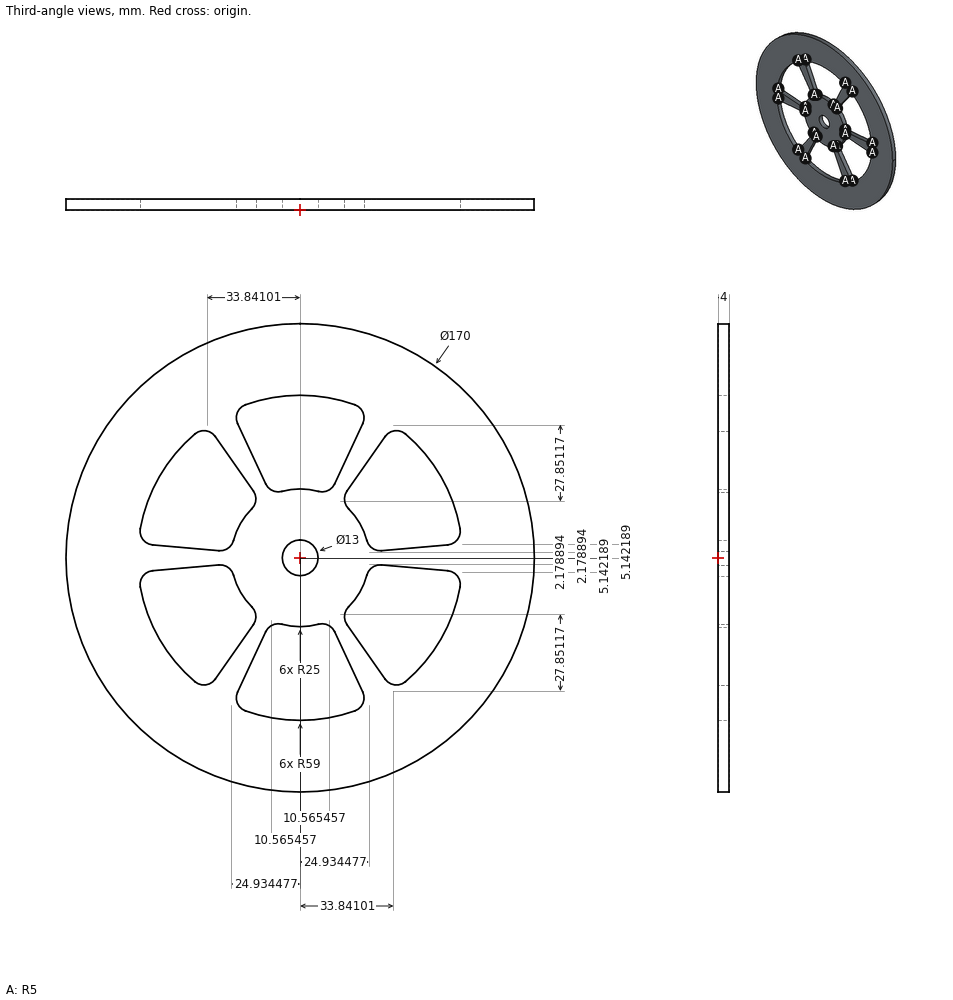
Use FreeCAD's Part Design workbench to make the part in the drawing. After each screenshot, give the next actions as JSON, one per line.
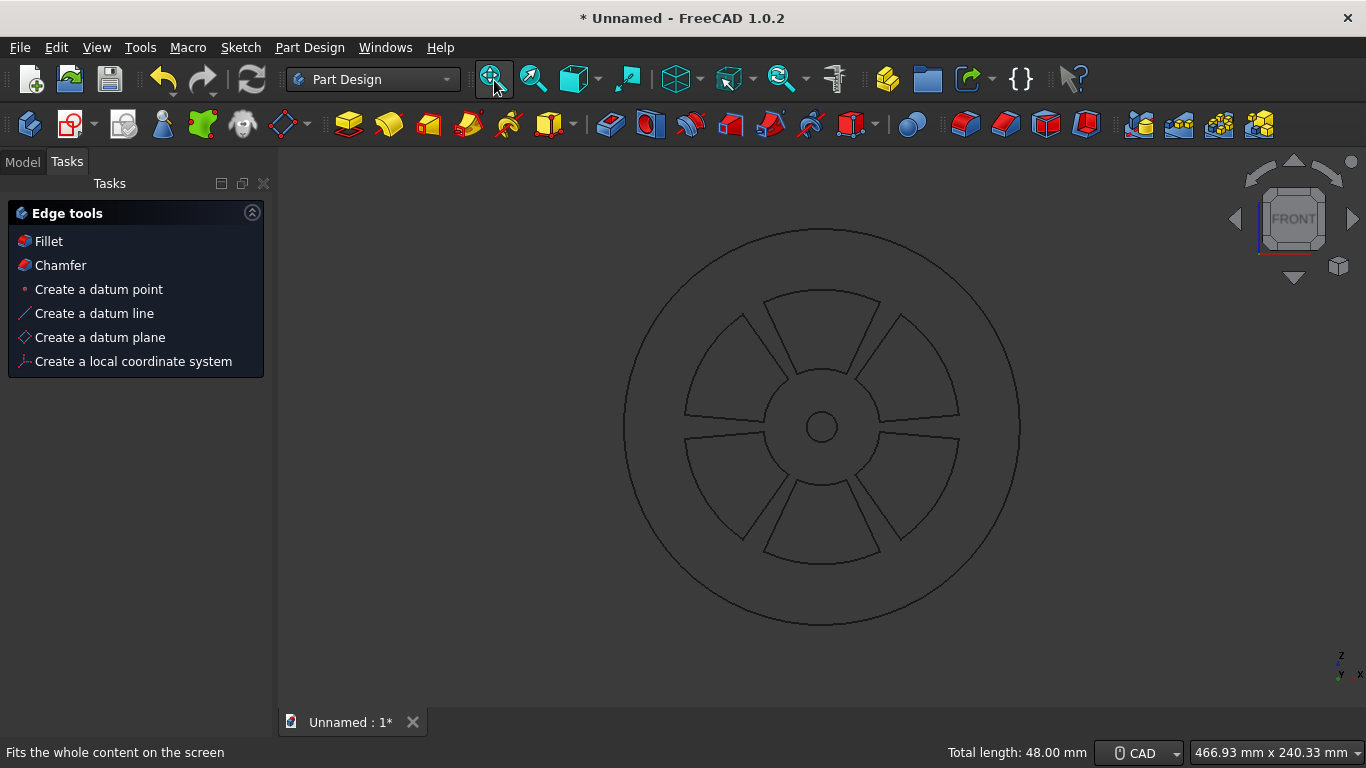
{"action": "scroll", "coordinate": [880, 421], "scroll_direction": "up", "scroll_amount": 8}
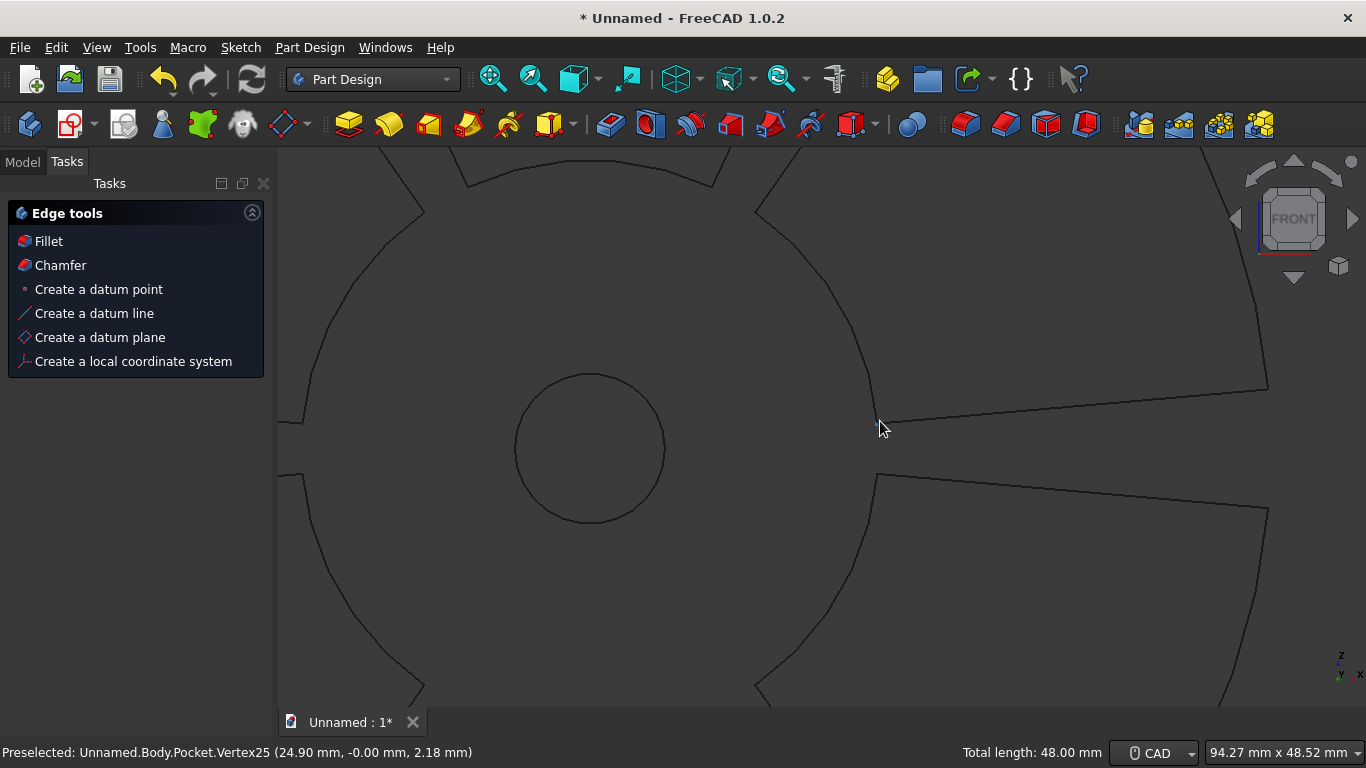
{"action": "left_click", "coordinate": [494, 80]}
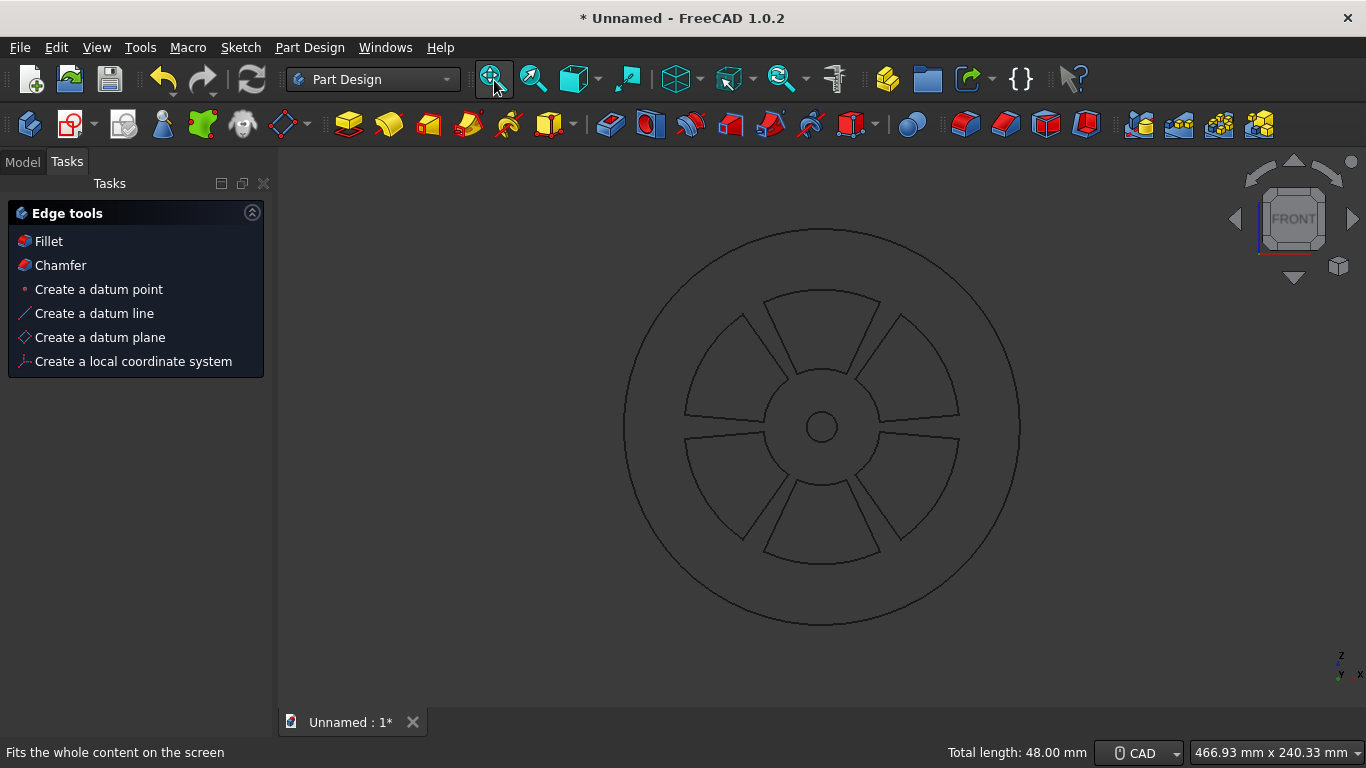
{"action": "key", "text": "3"}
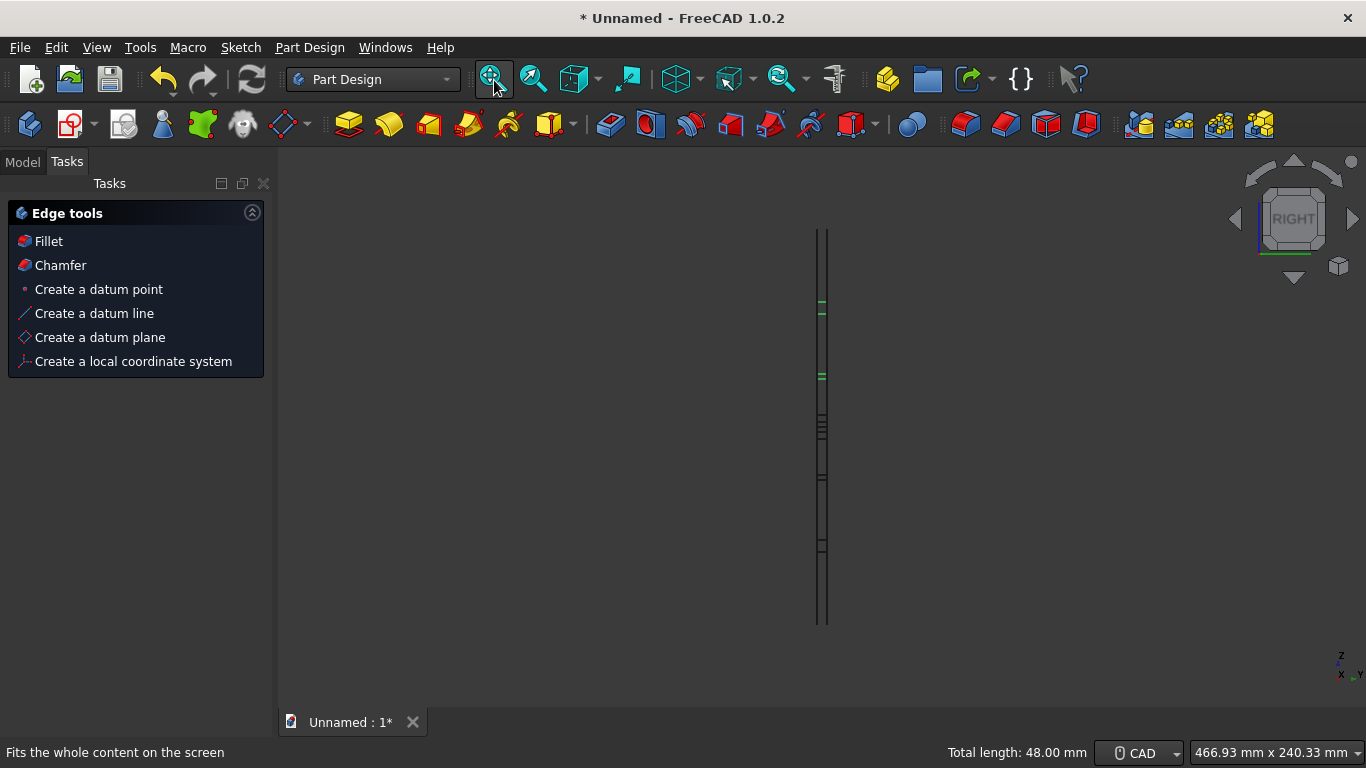
{"action": "scroll", "coordinate": [822, 421], "scroll_direction": "up", "scroll_amount": 8}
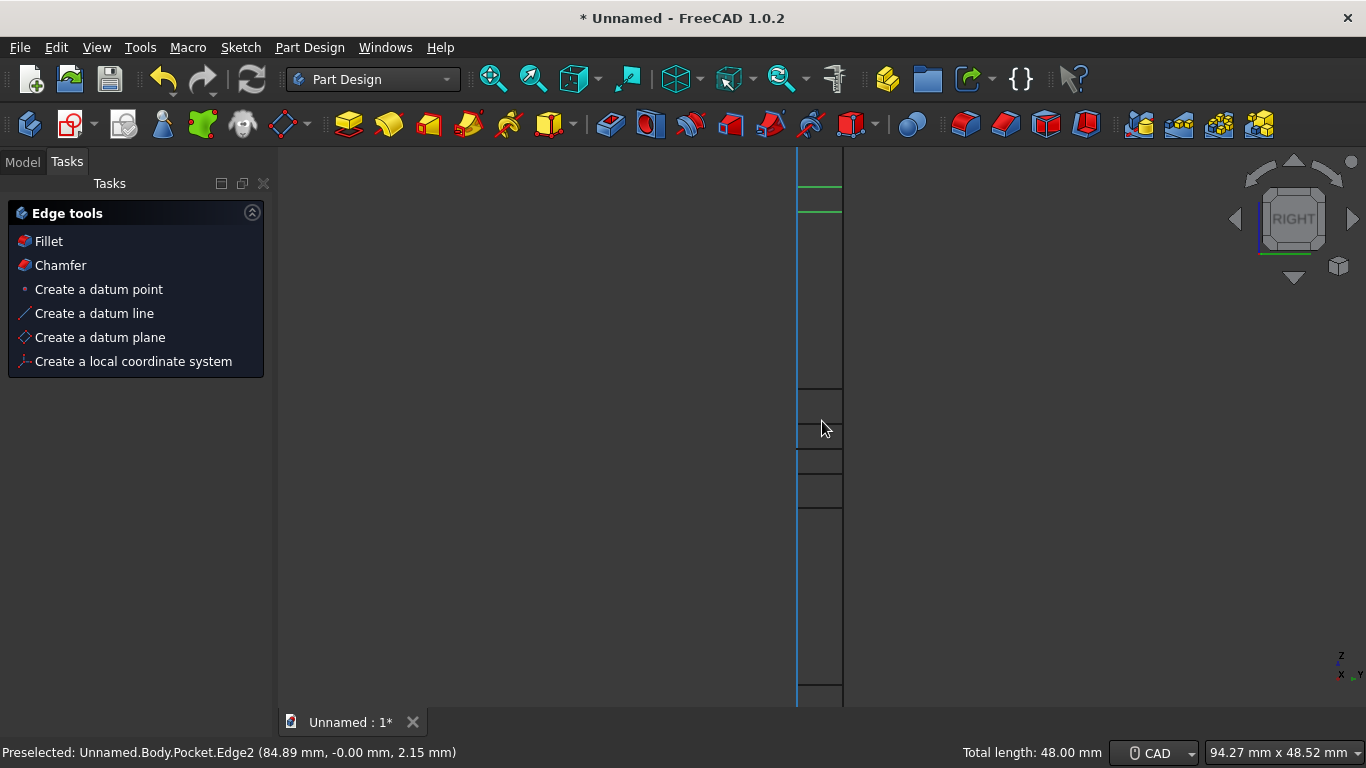
{"action": "left_click", "coordinate": [820, 423], "text": "ctrl"}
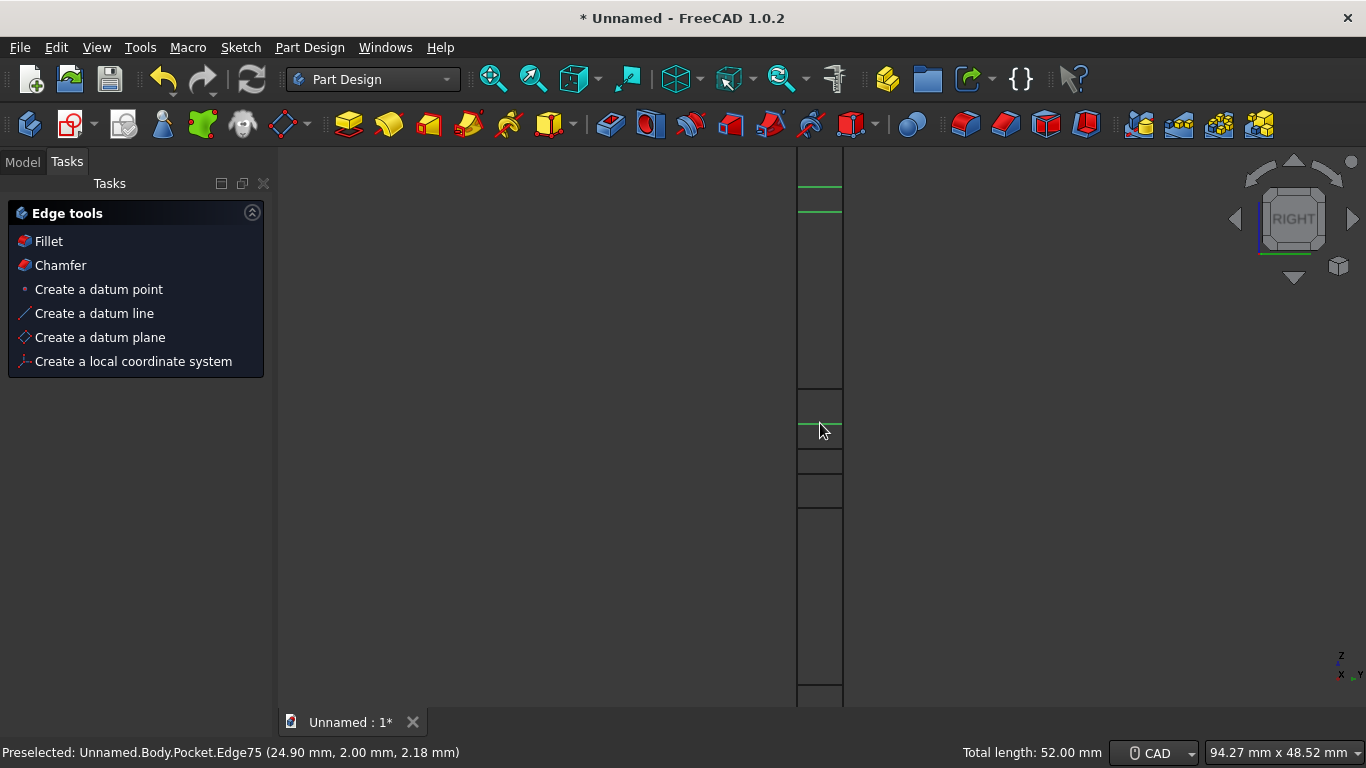
{"action": "left_click", "coordinate": [820, 388], "text": "ctrl"}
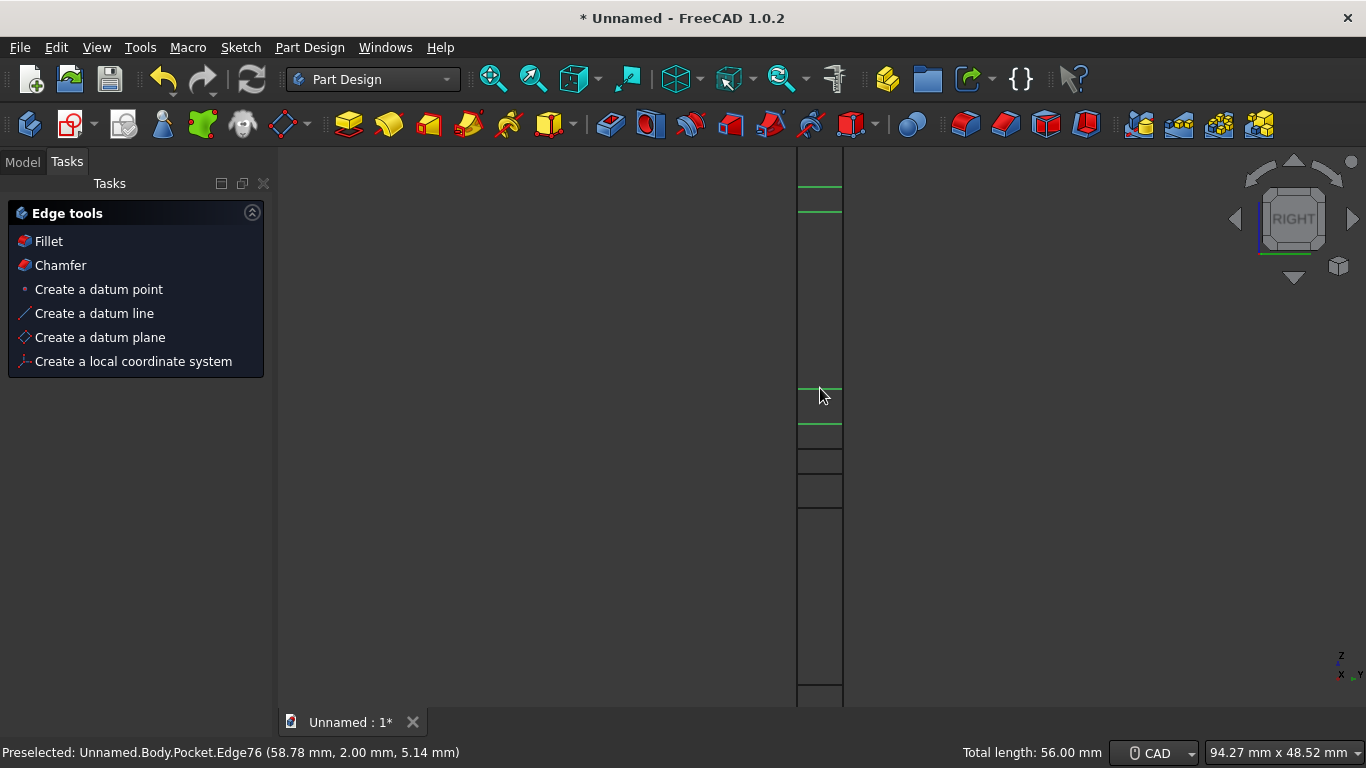
{"action": "left_click", "coordinate": [820, 473], "text": "ctrl"}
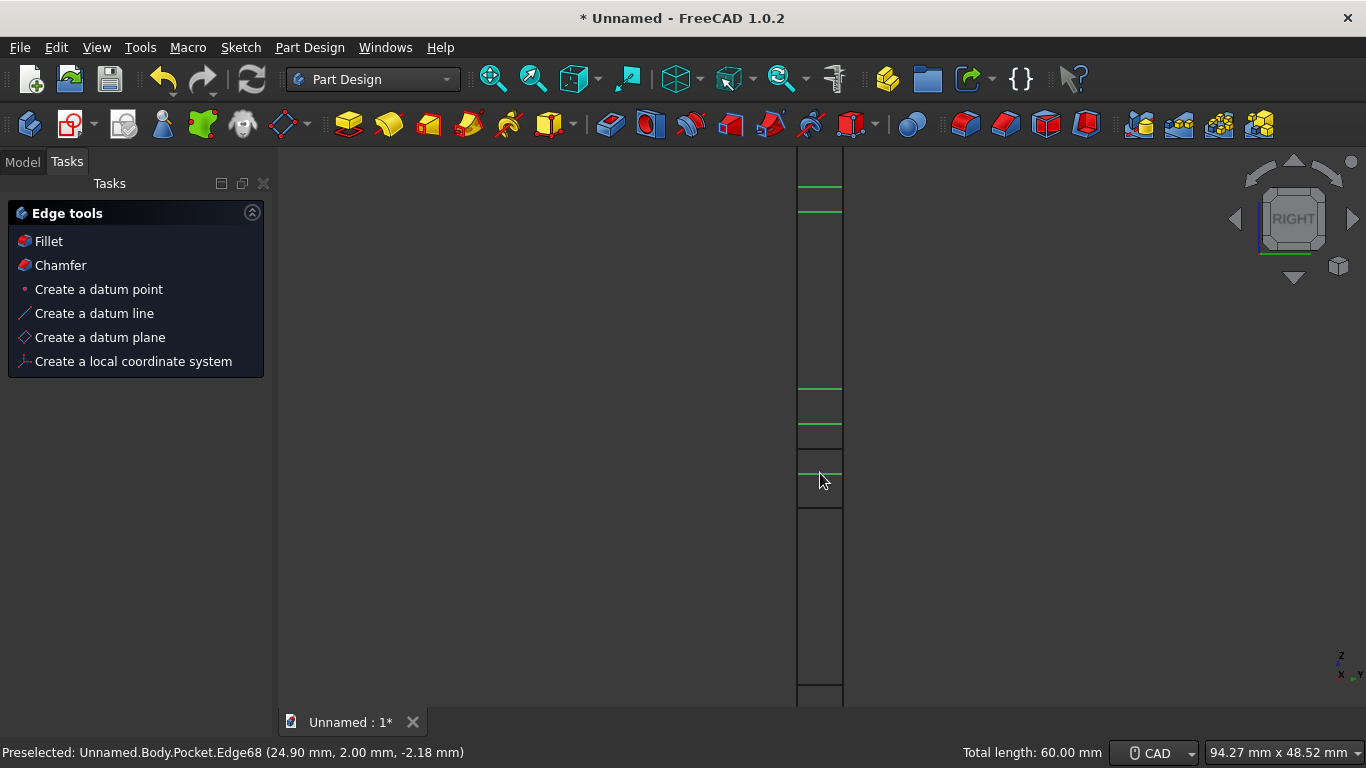
{"action": "left_click", "coordinate": [820, 507], "text": "ctrl"}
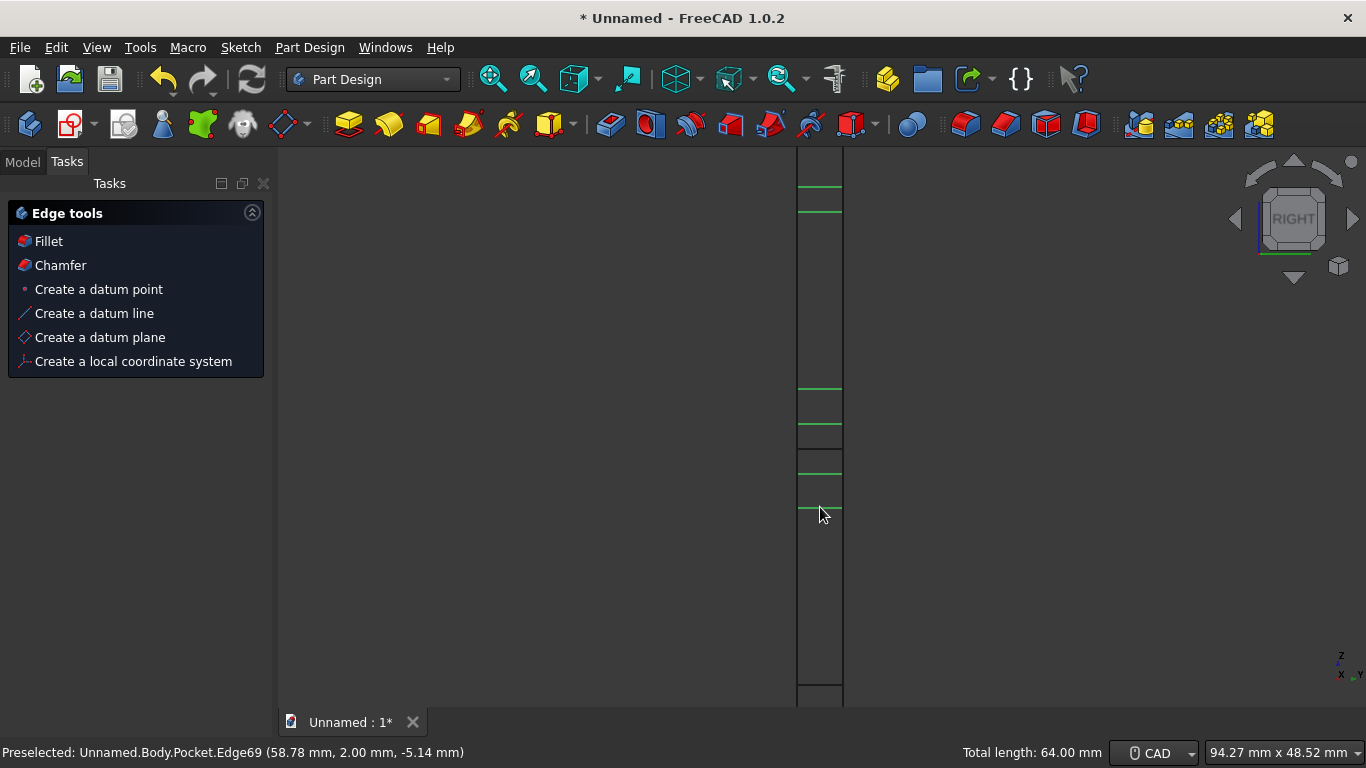
{"action": "left_click", "coordinate": [494, 80]}